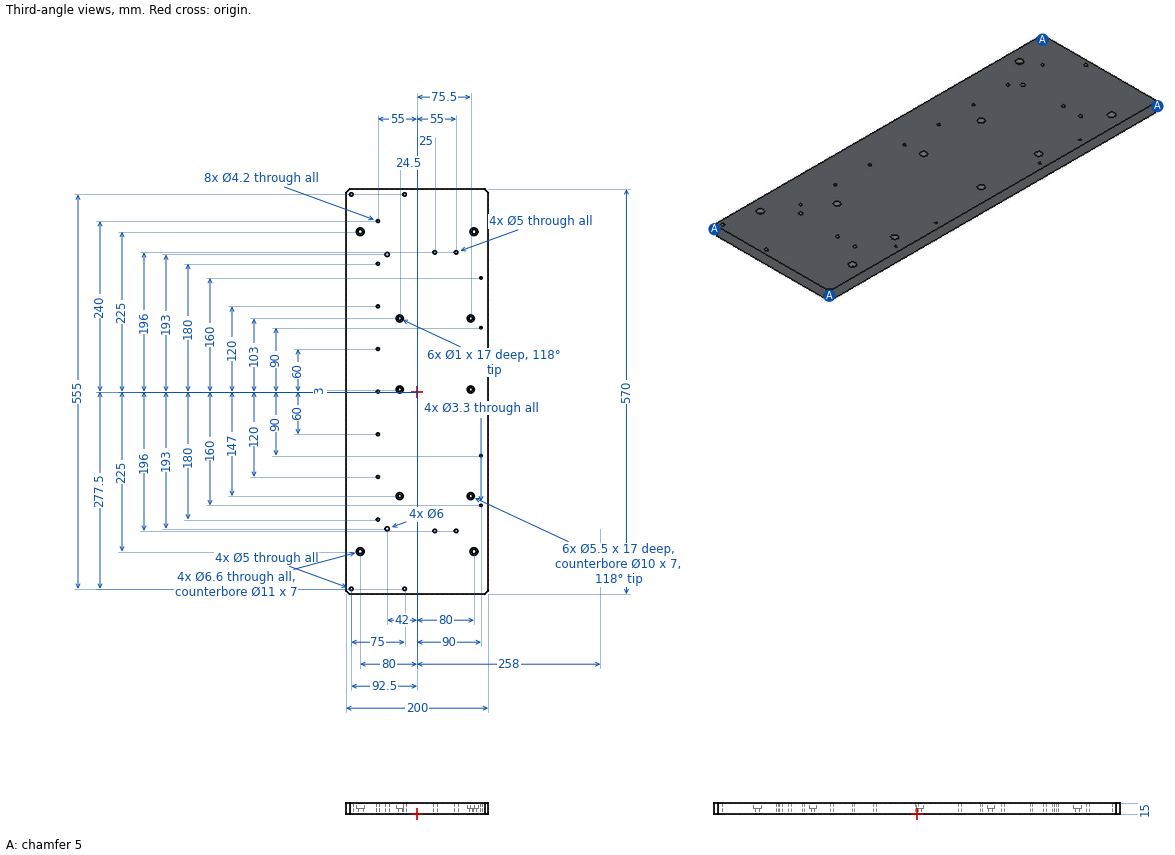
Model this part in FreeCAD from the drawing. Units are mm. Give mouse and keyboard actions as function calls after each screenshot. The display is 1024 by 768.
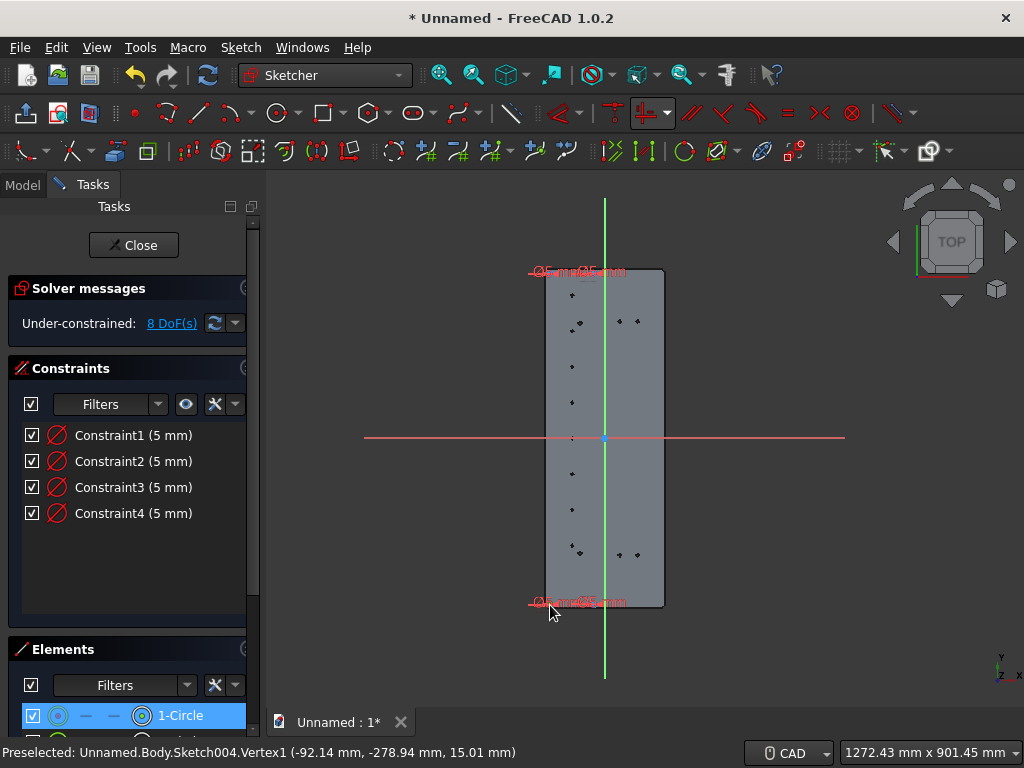
click(594, 604)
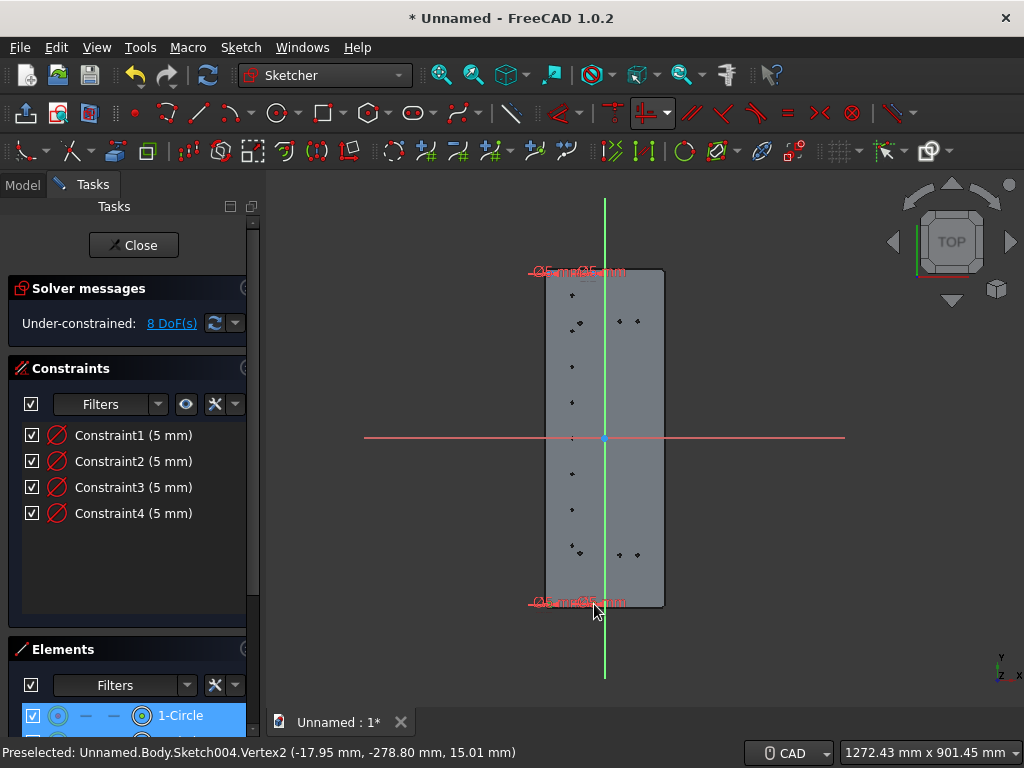
click(670, 114)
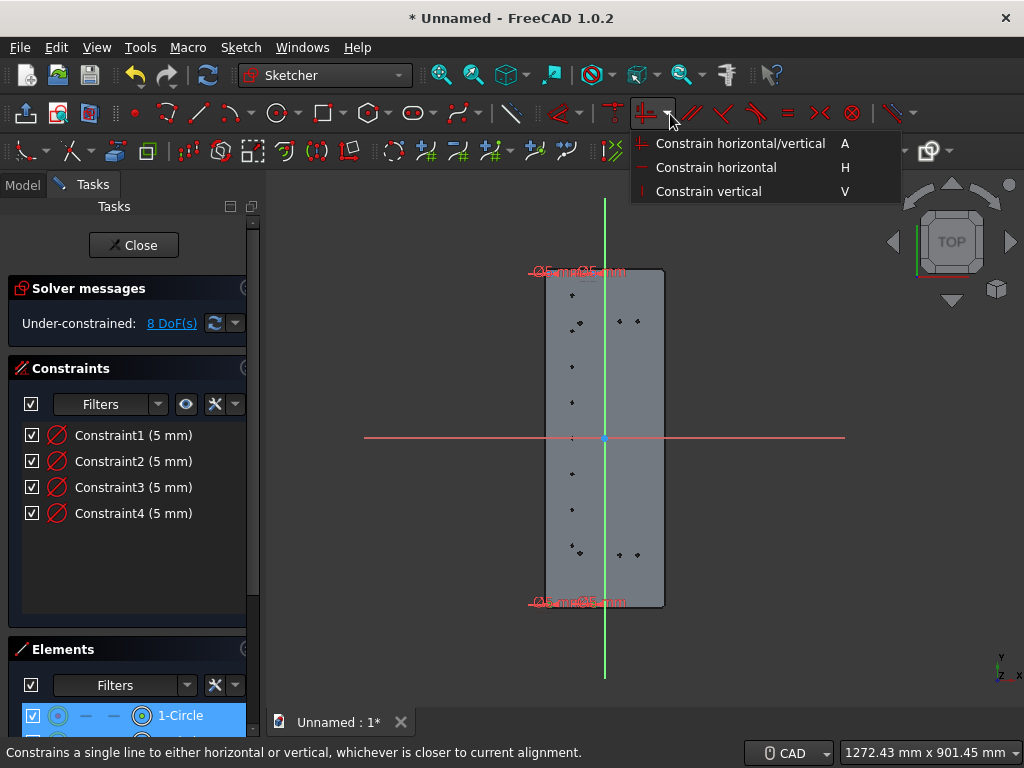
click(766, 167)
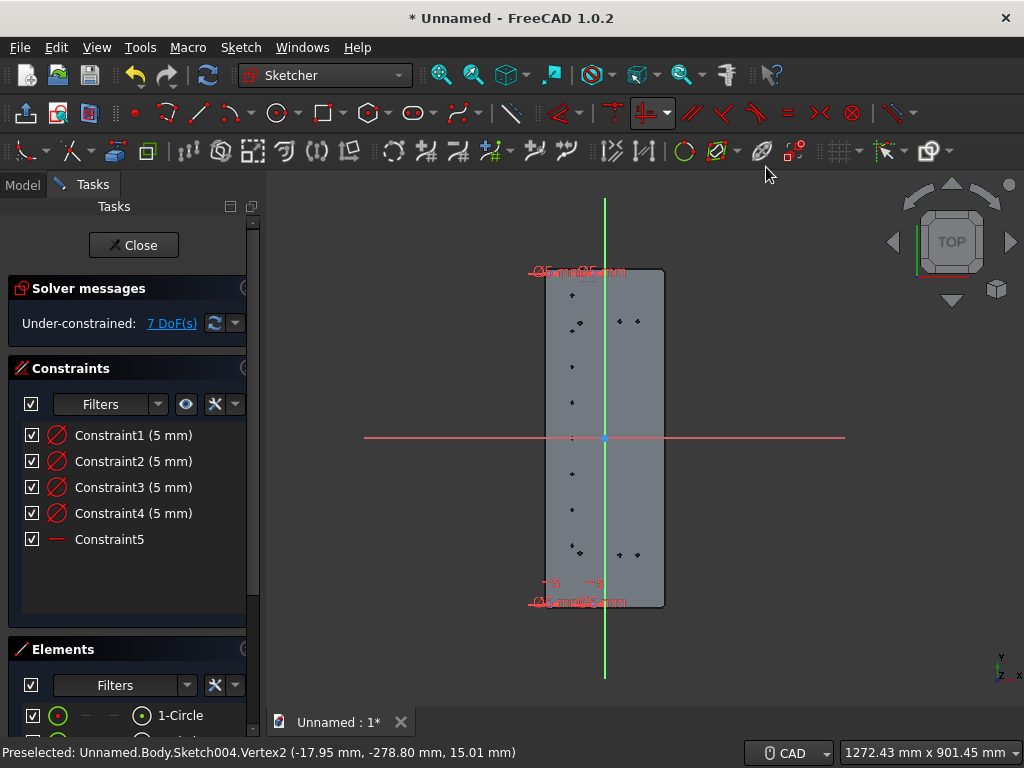
click(594, 605)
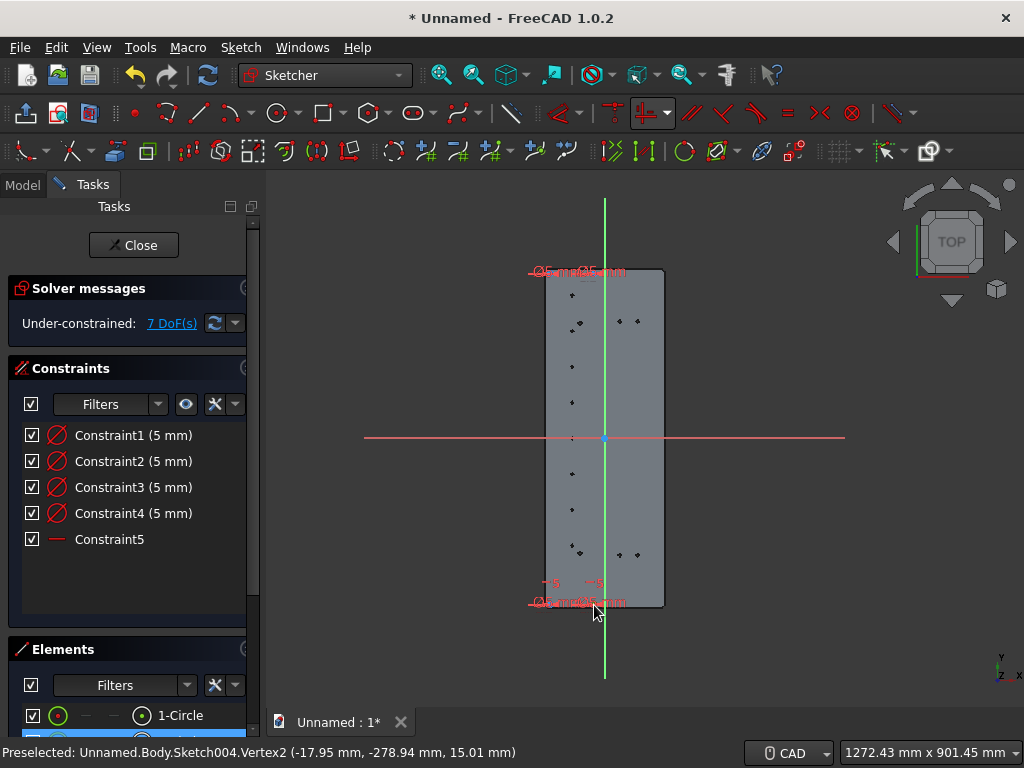
click(594, 274)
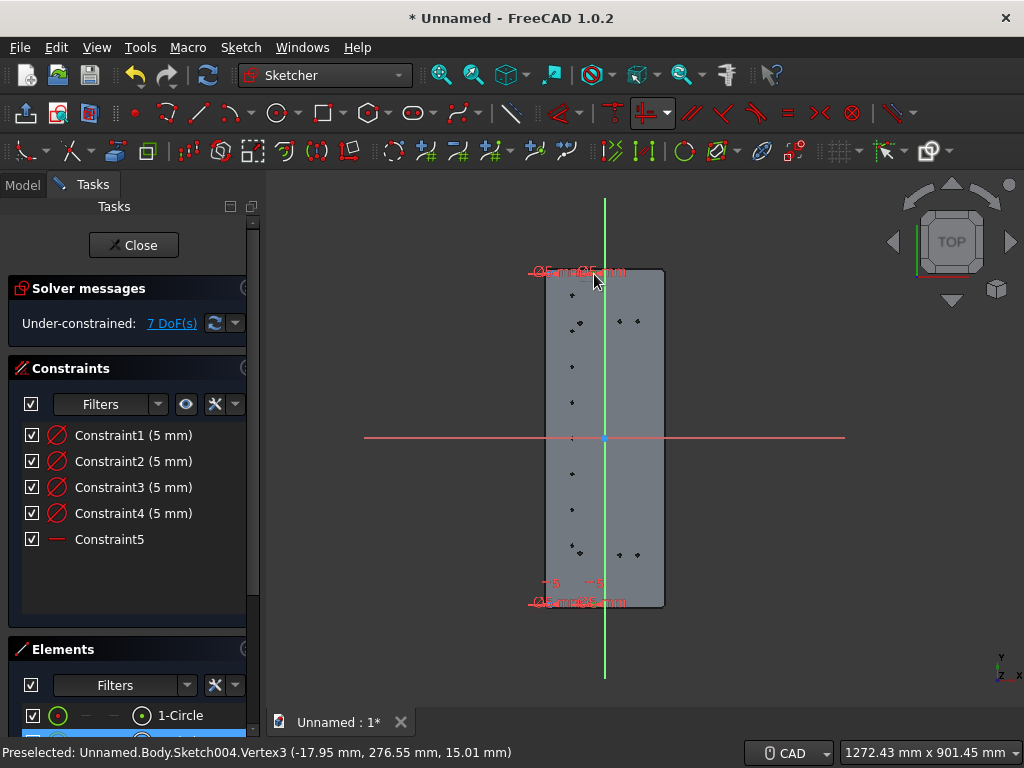
key(v)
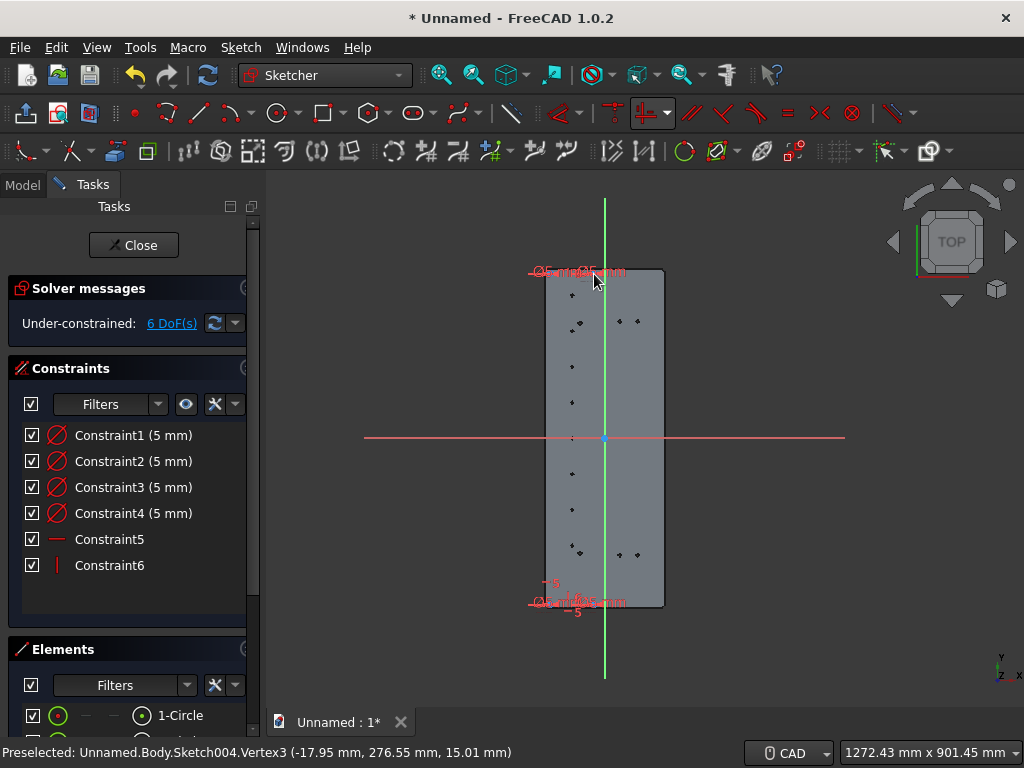
click(550, 605)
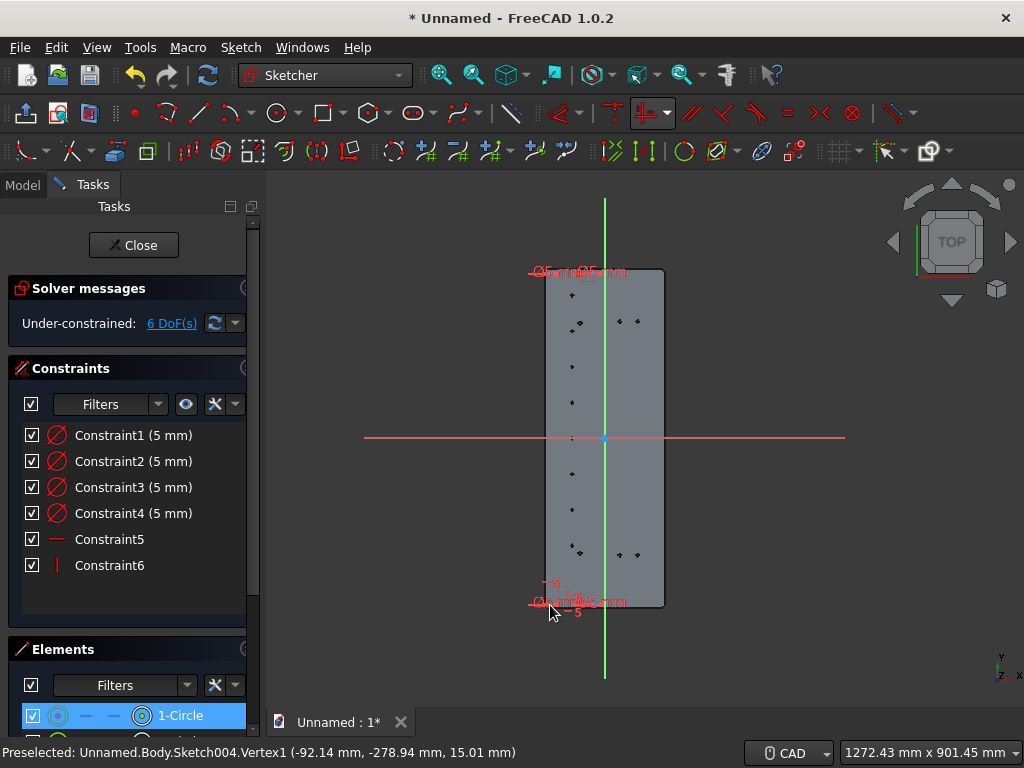
click(550, 274)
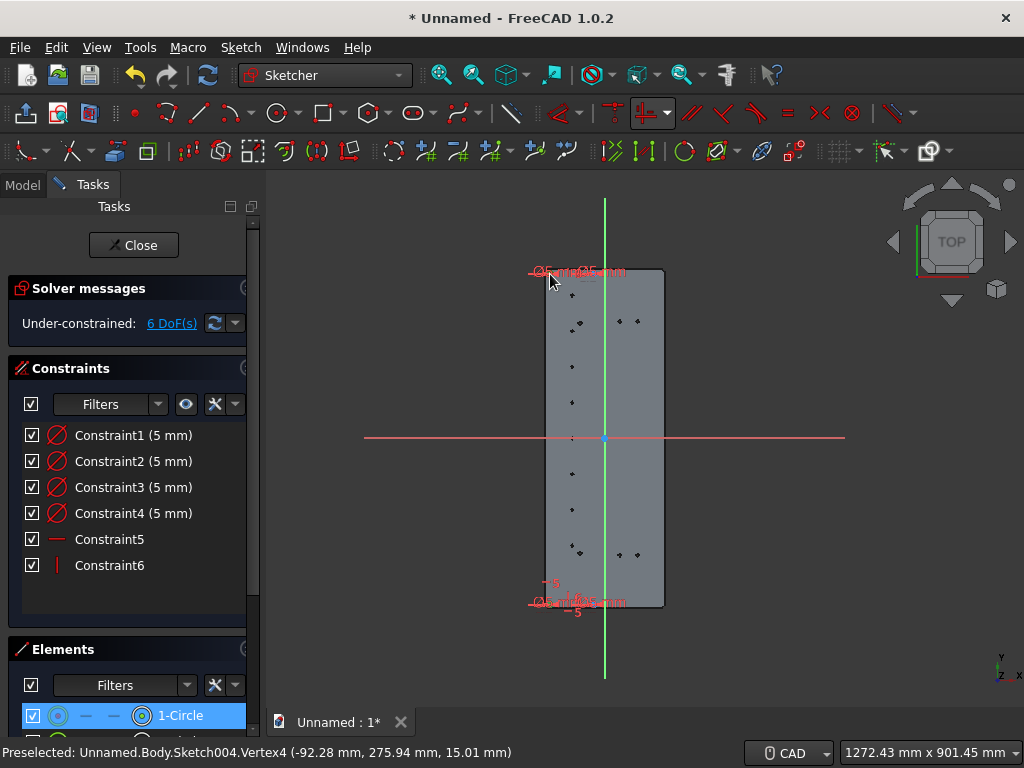
key(v)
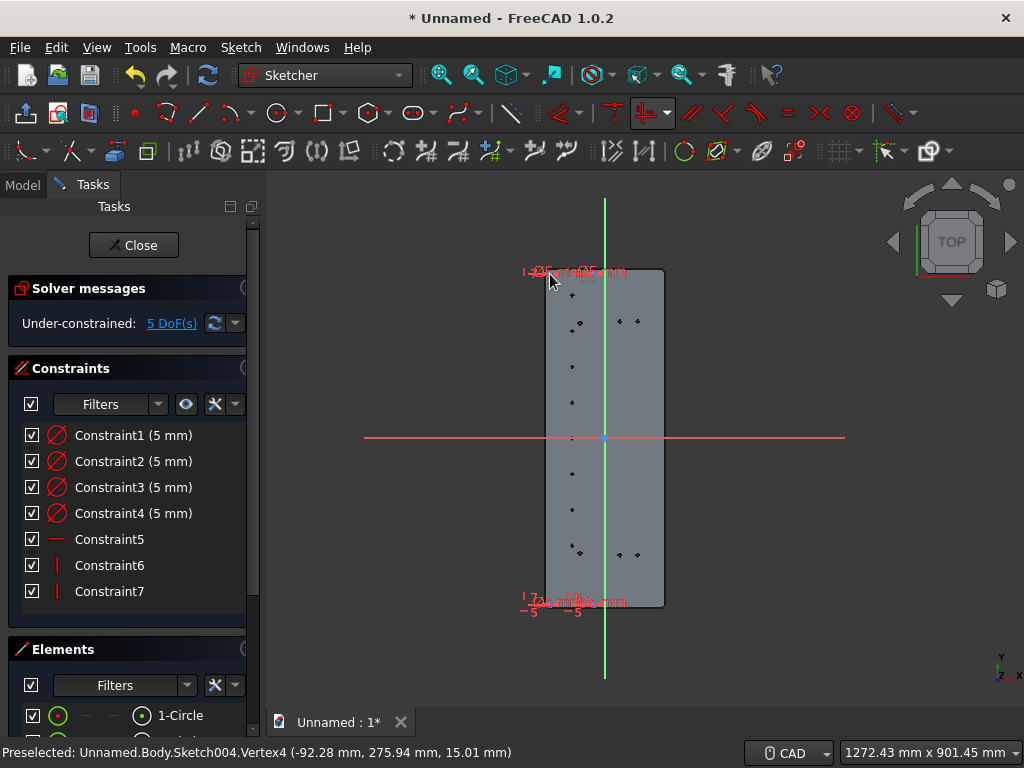
click(594, 274)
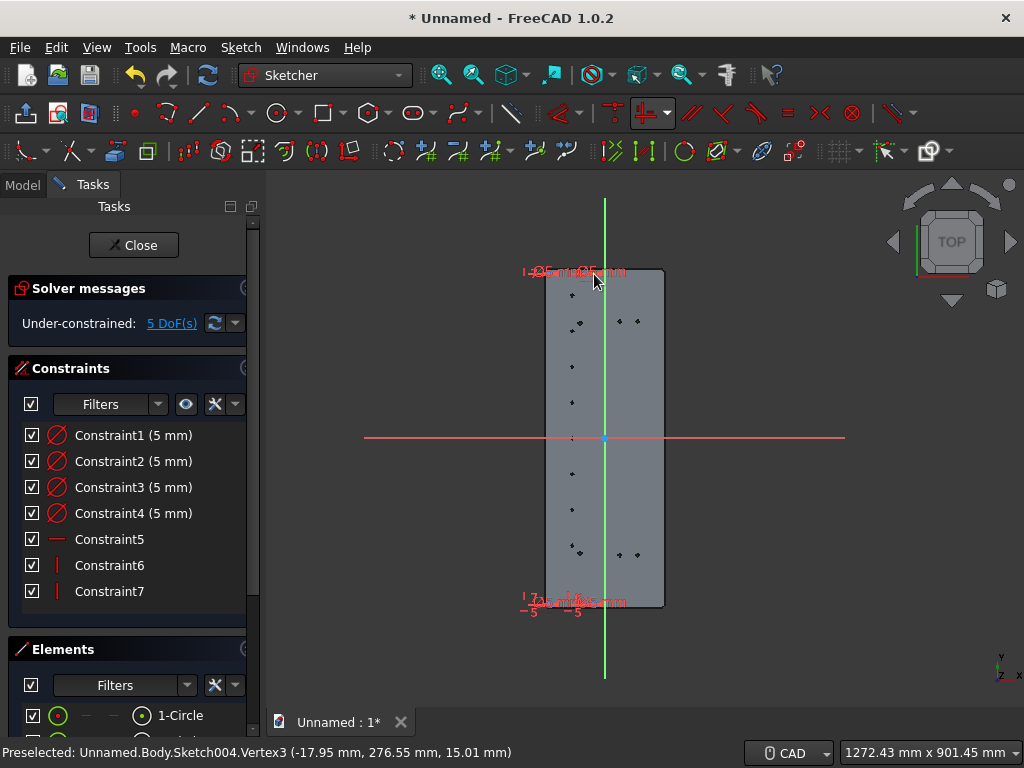
click(550, 274)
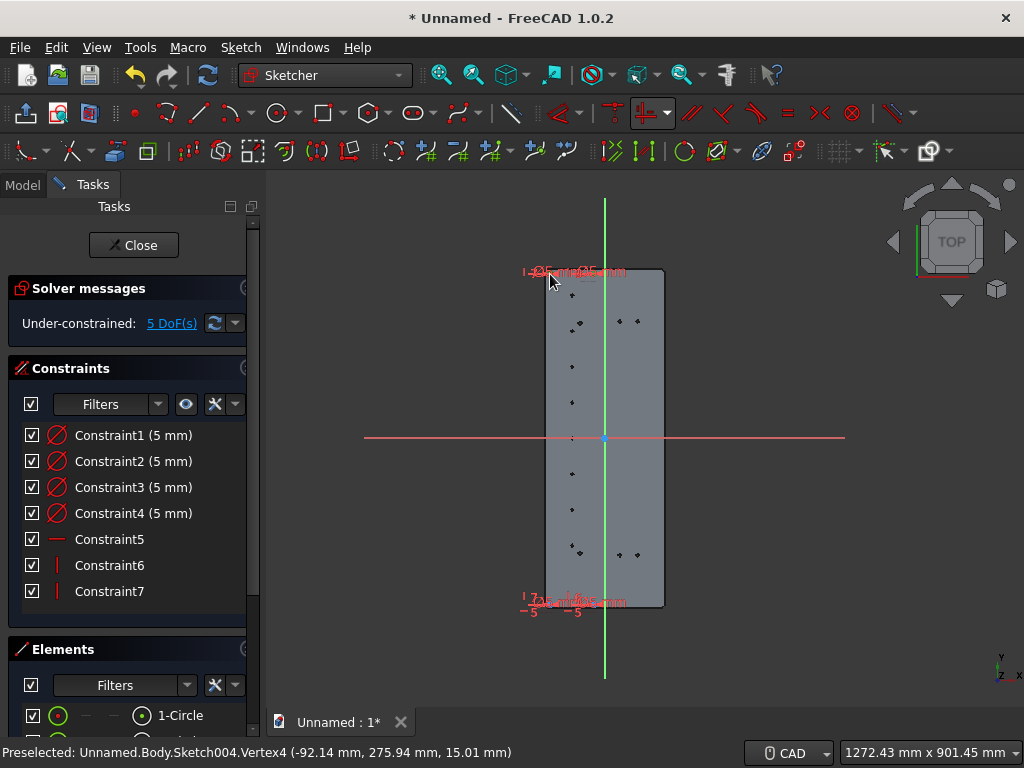
click(670, 114)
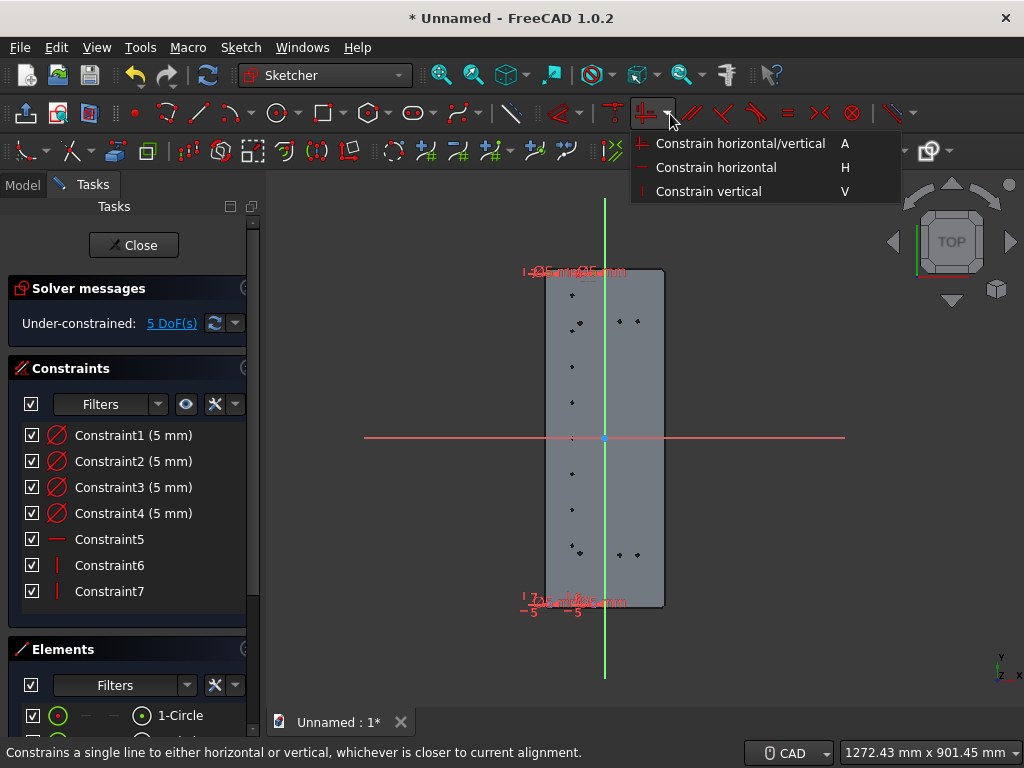
click(766, 167)